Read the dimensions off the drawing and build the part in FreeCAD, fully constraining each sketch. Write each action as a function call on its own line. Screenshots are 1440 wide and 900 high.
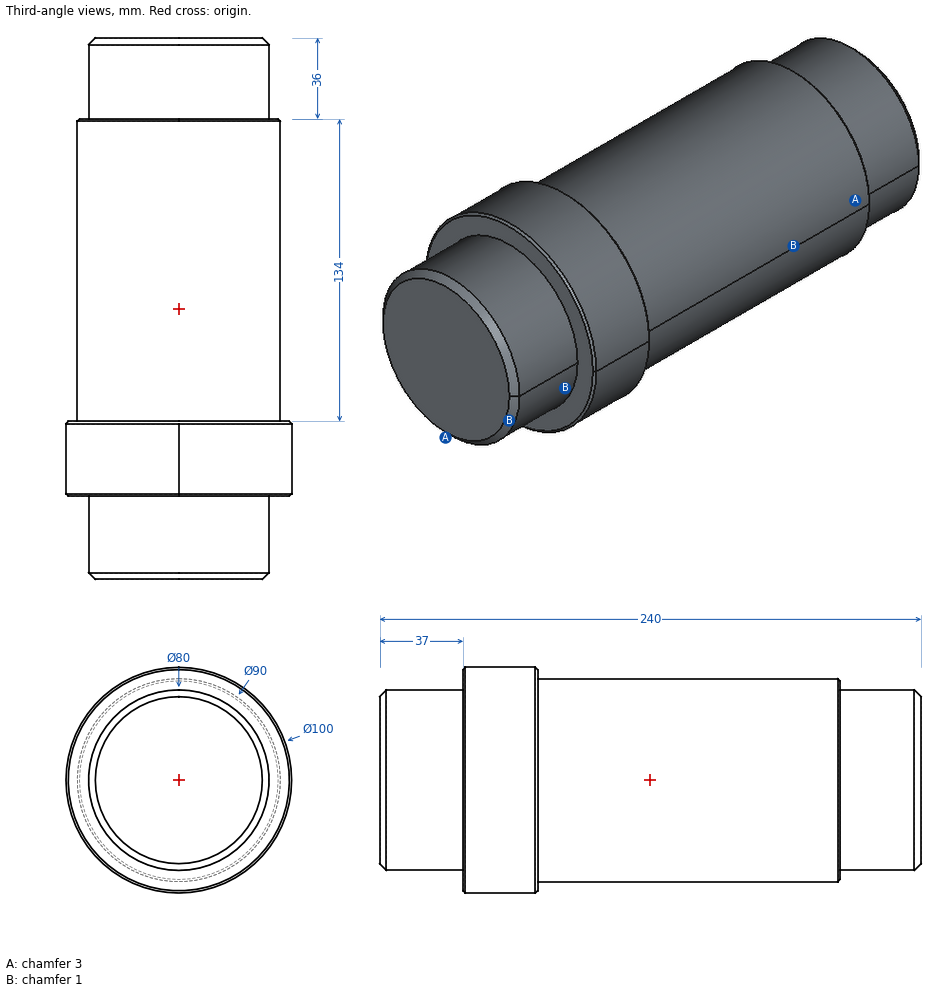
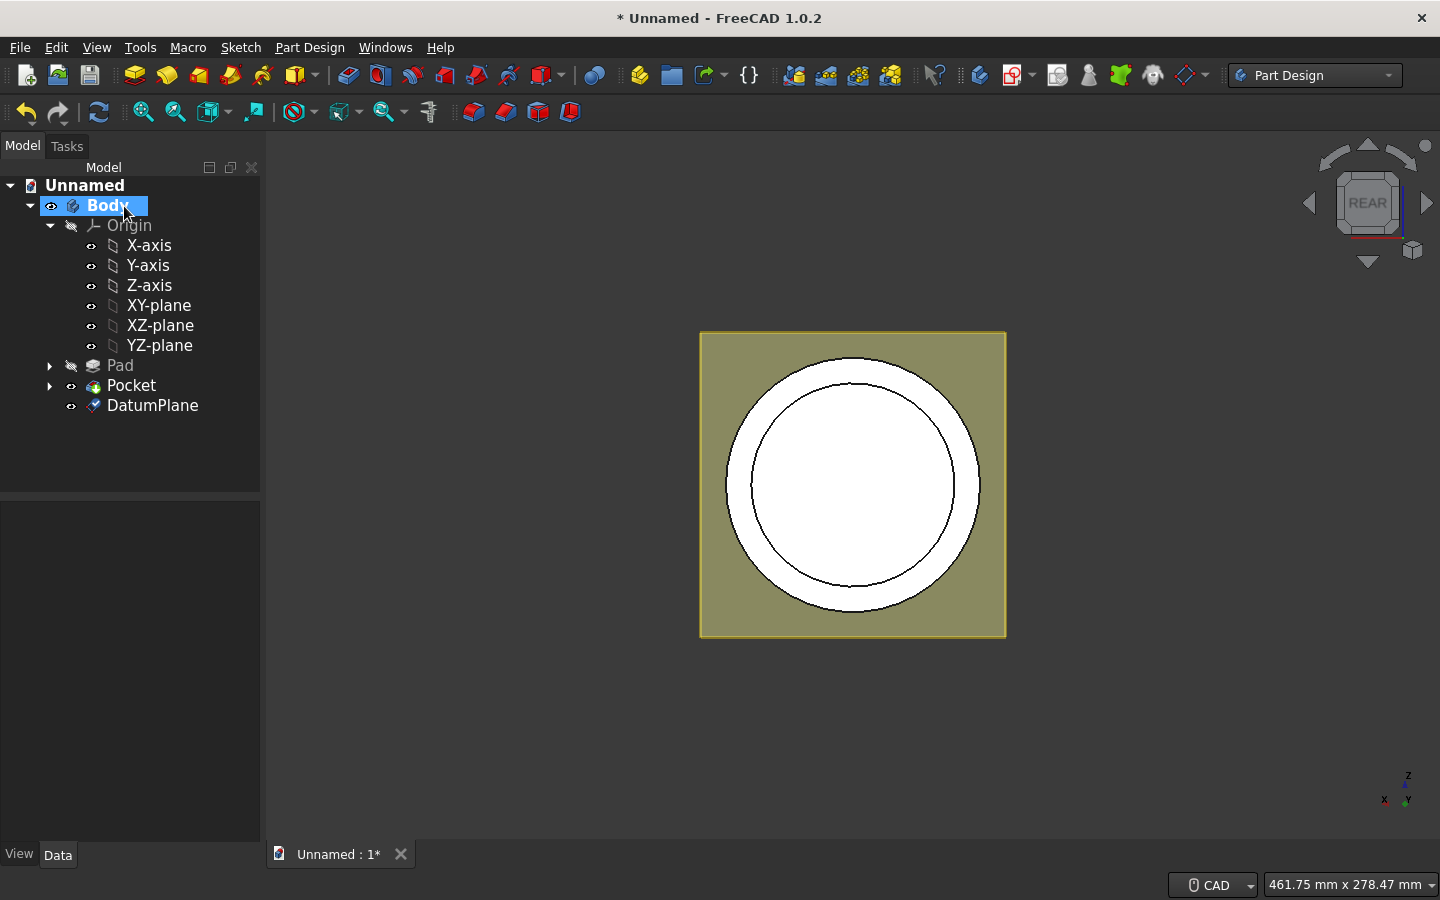
click(116, 406)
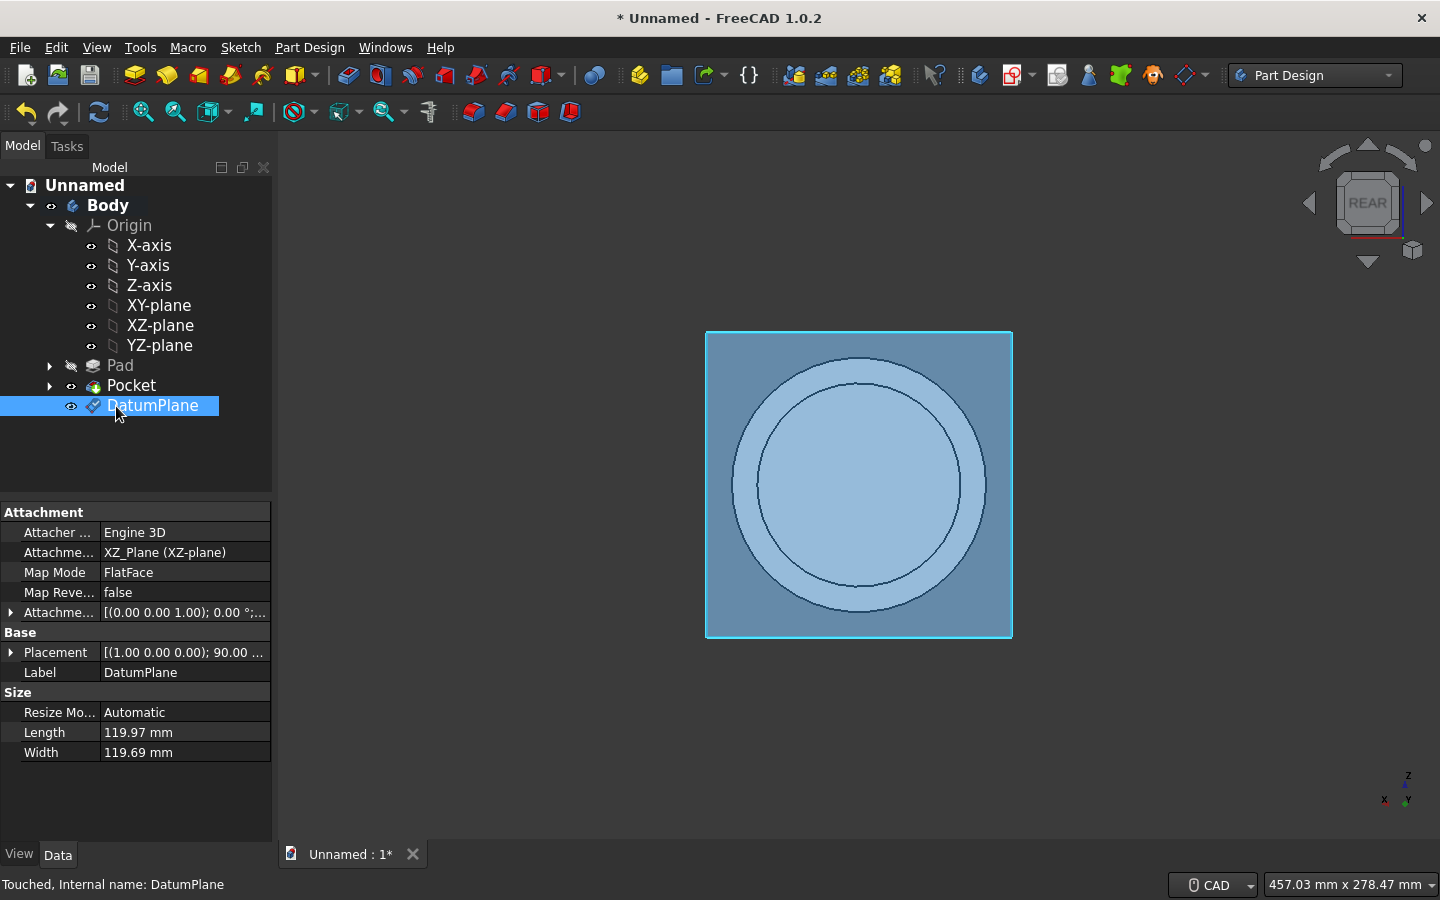
click(1012, 76)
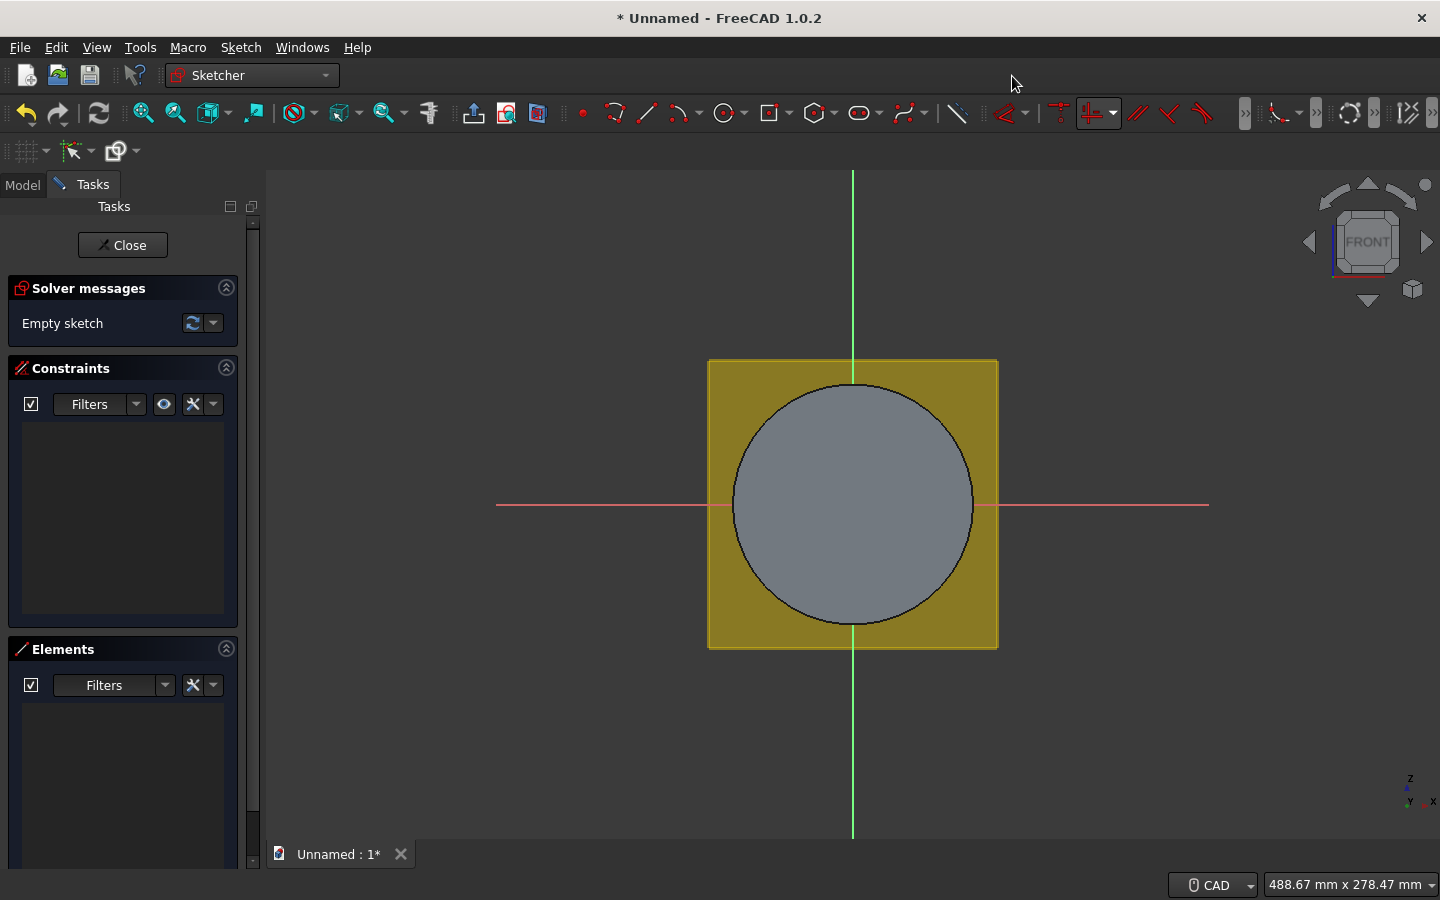
click(538, 114)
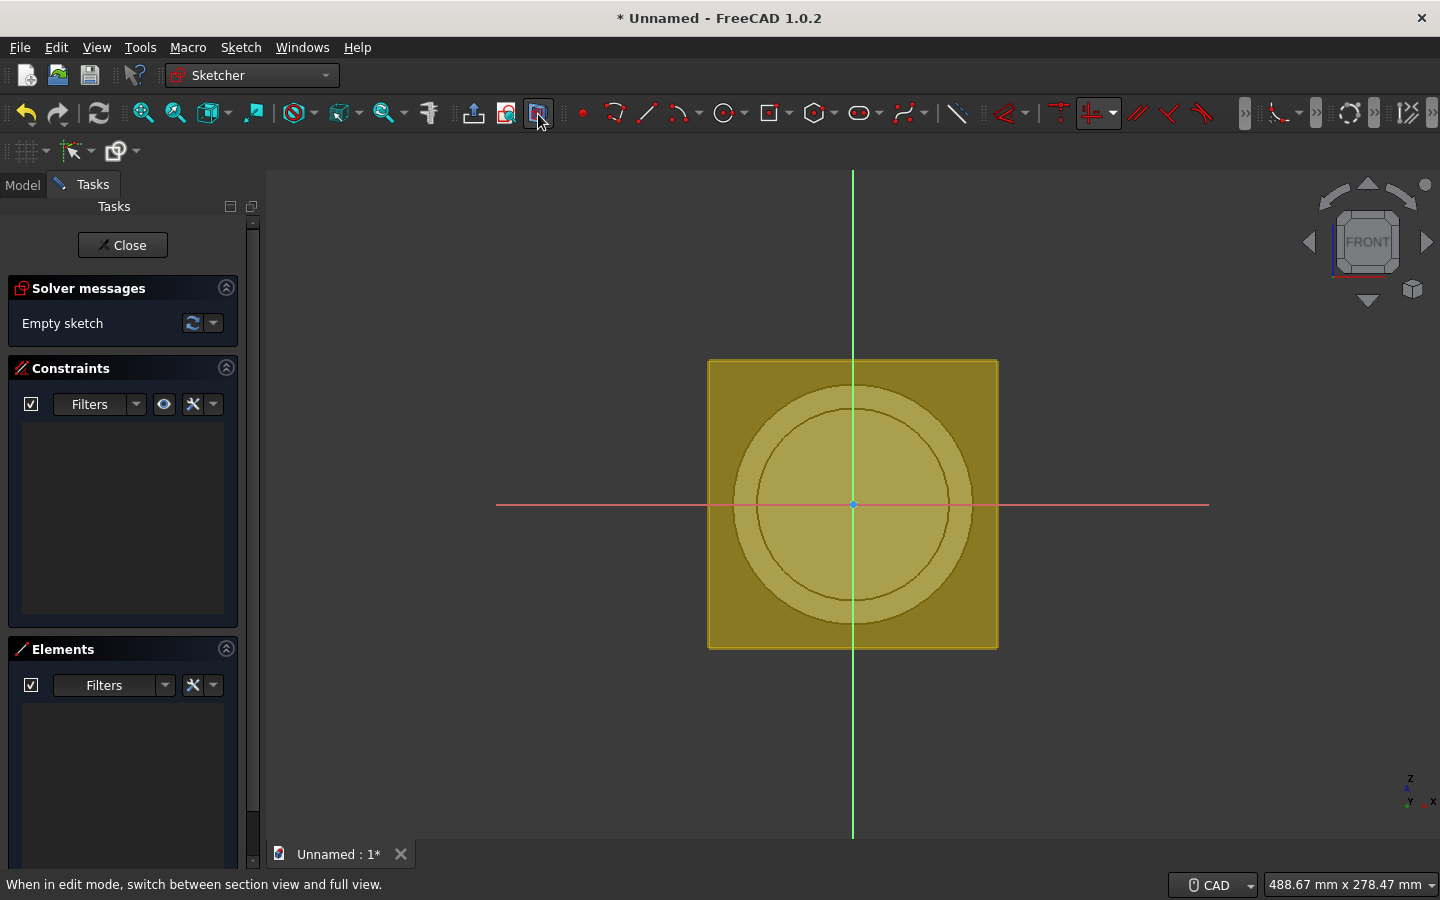
scroll(936, 504, up, 3)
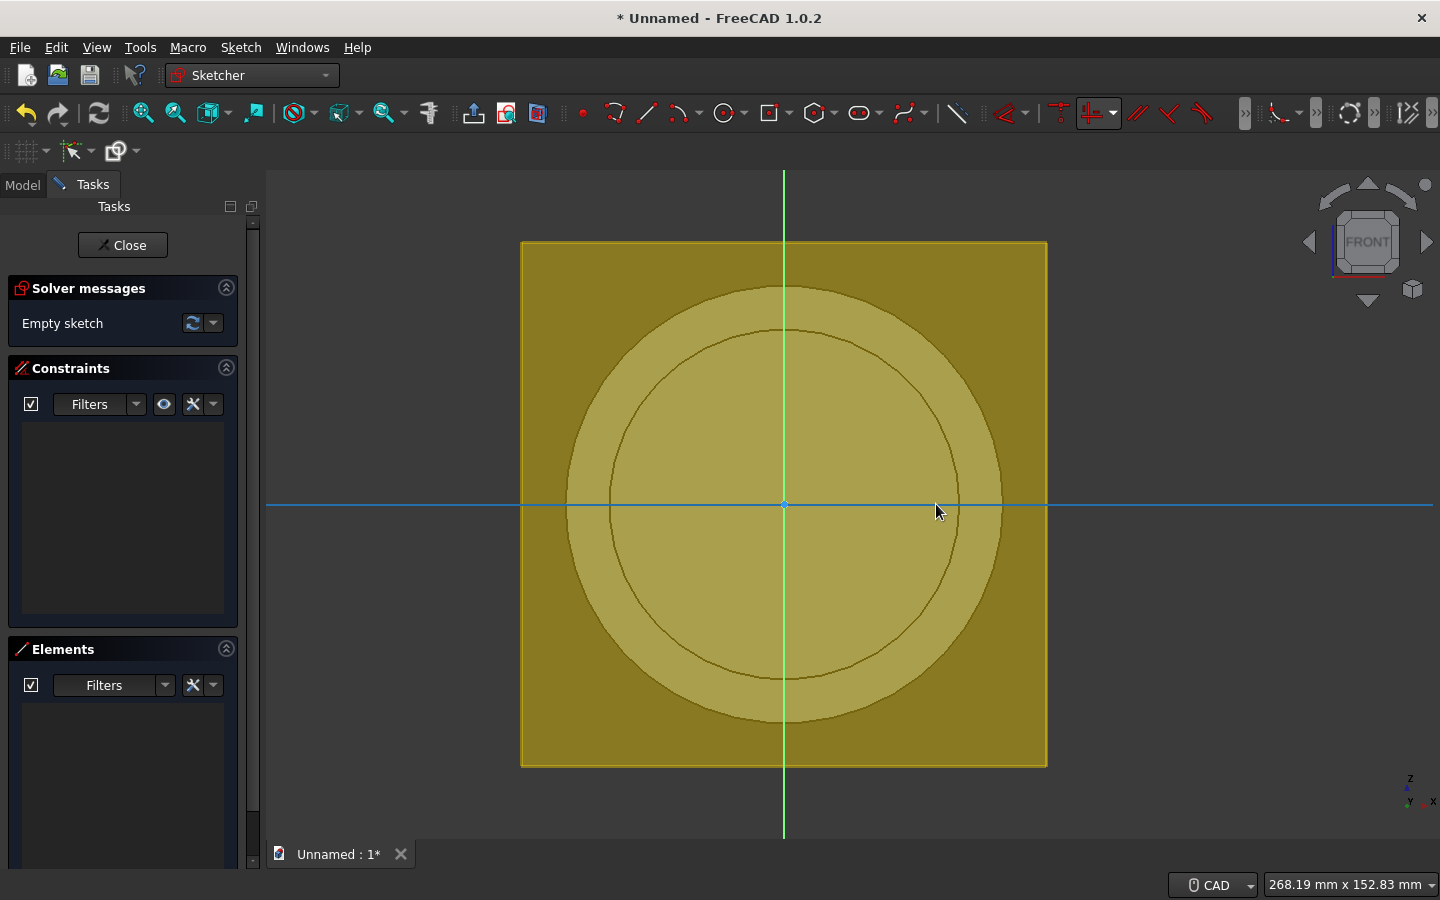
click(724, 114)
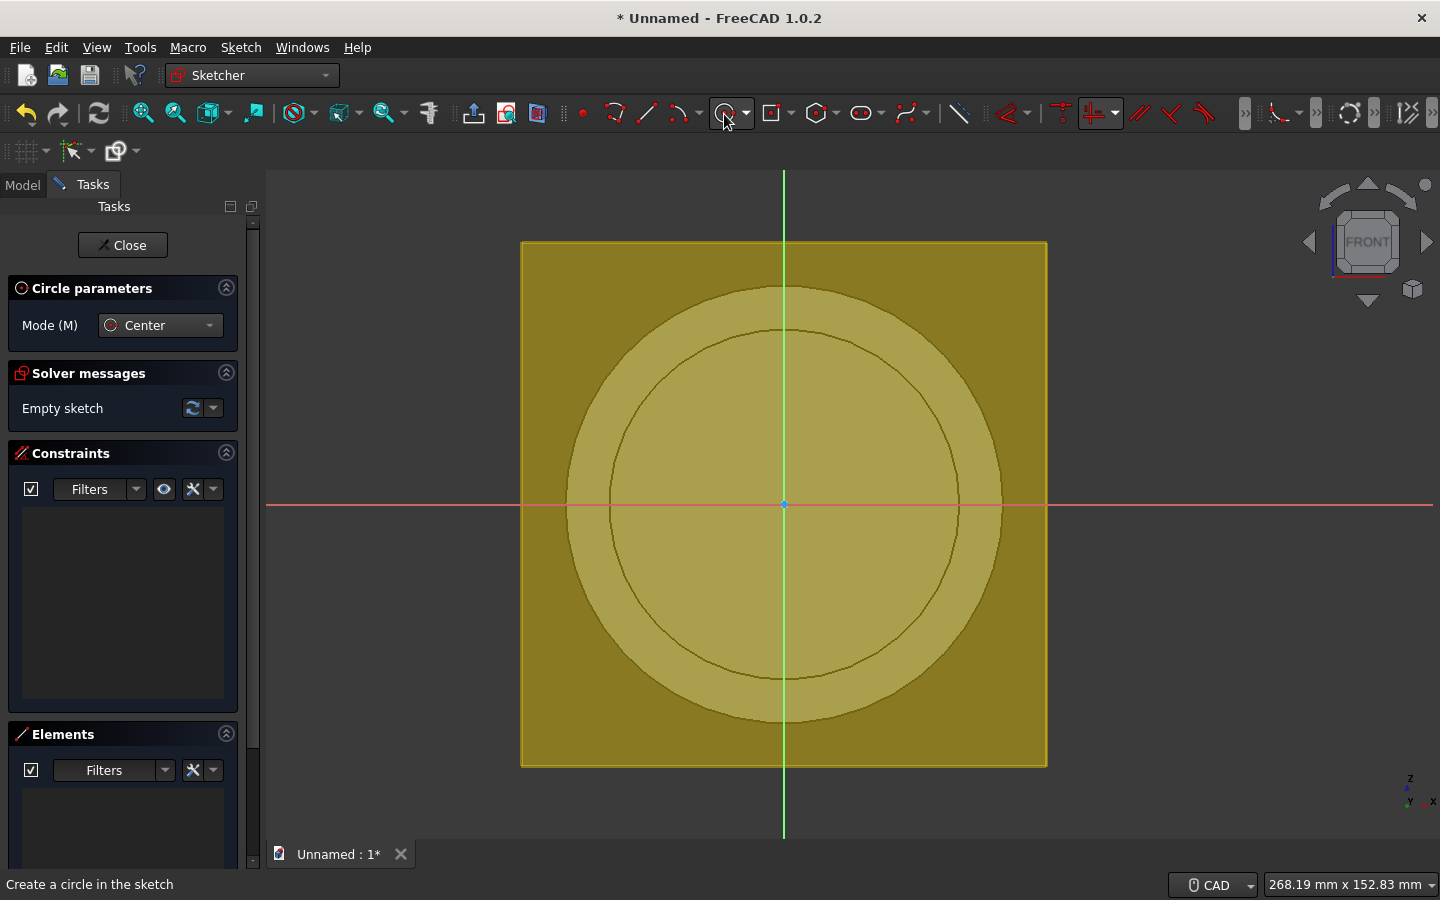
click(784, 504)
click(939, 350)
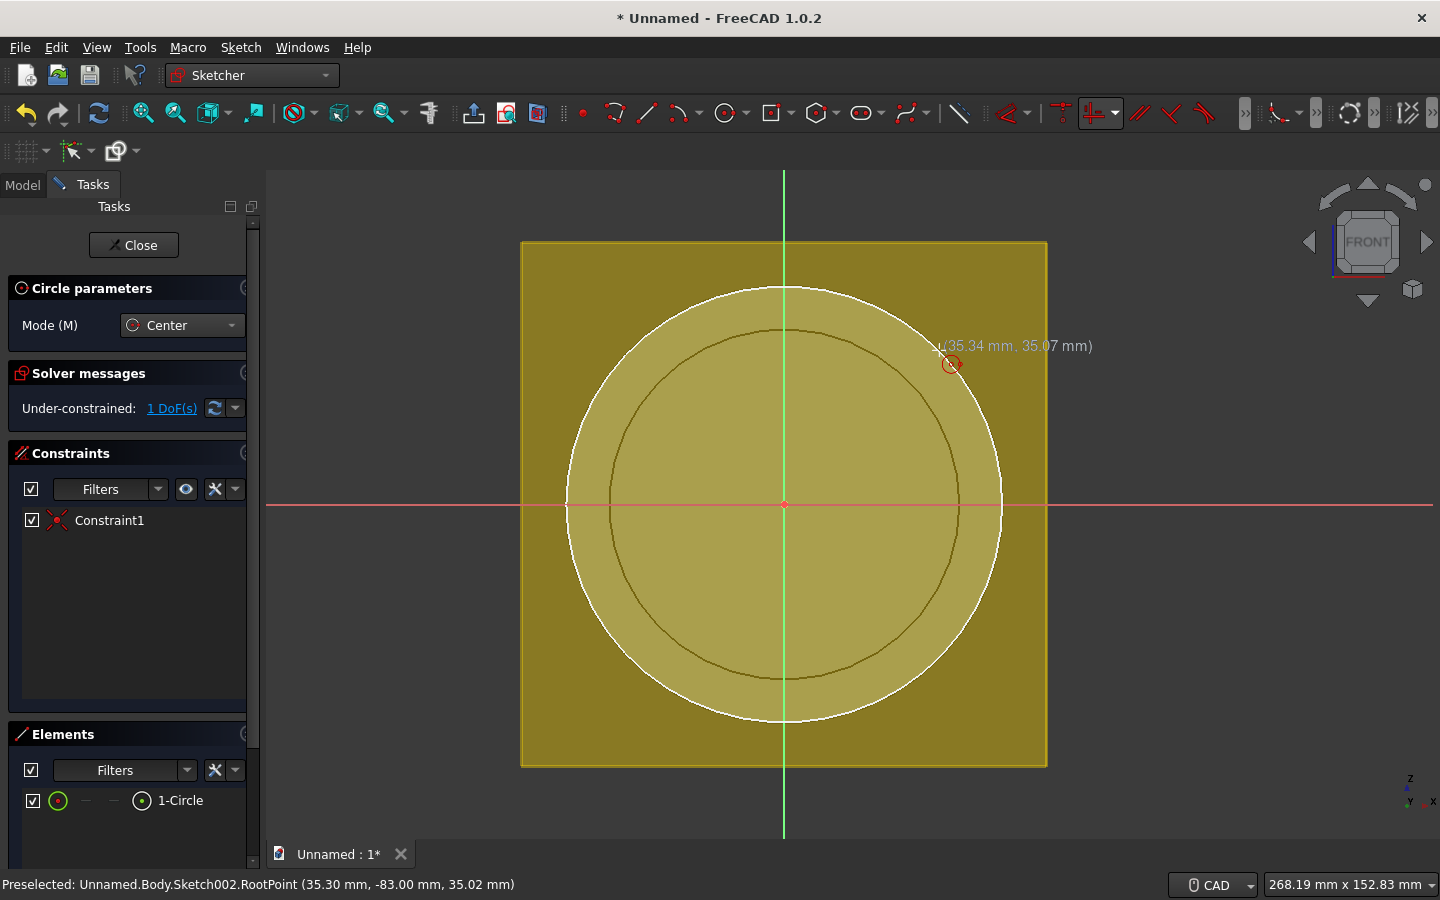
click(784, 504)
click(908, 381)
key(Escape)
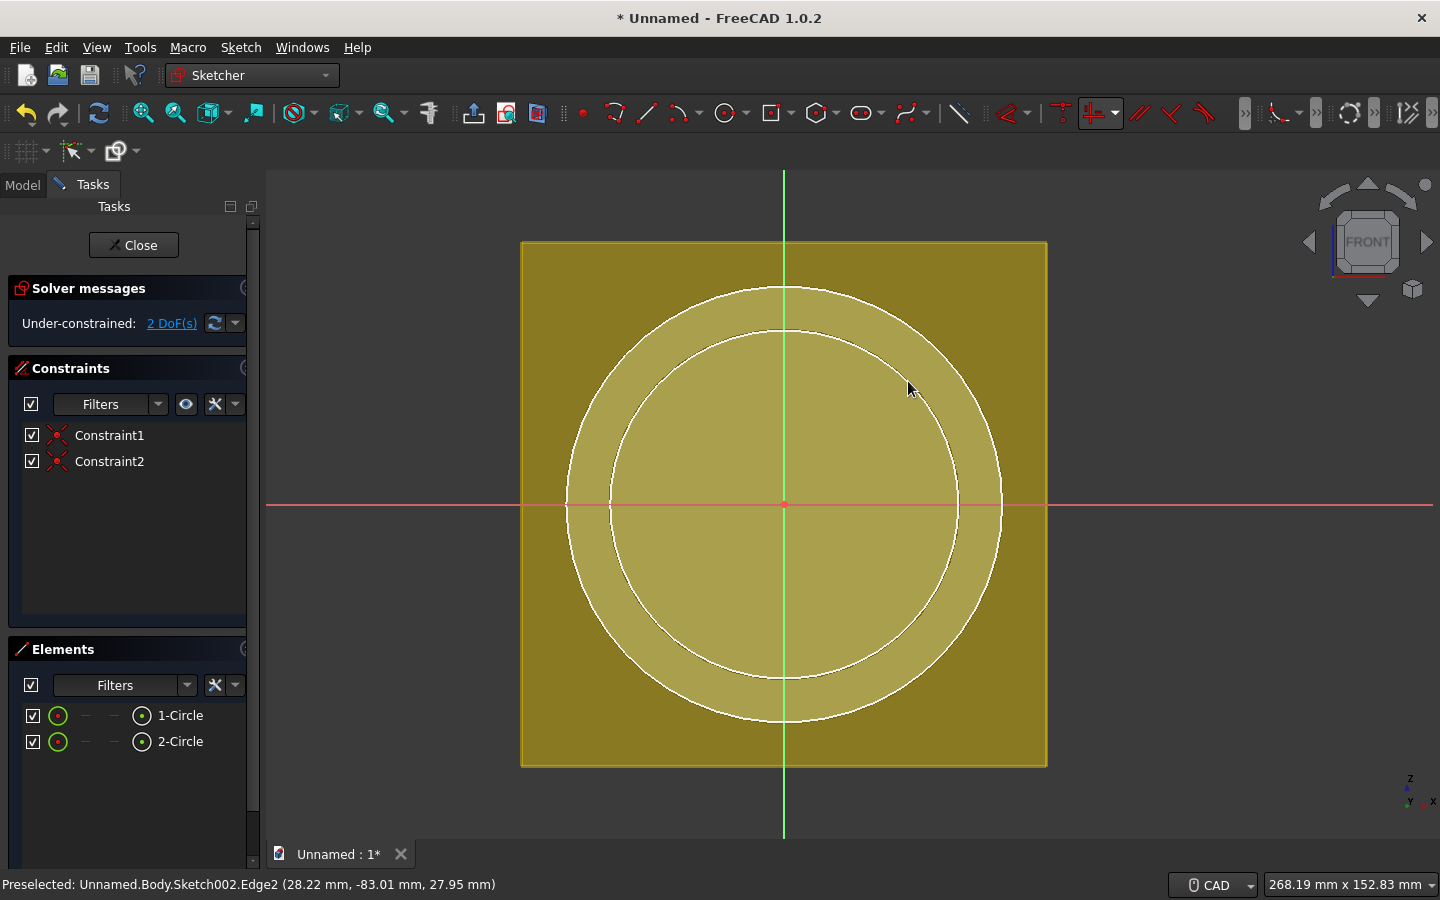
click(1006, 114)